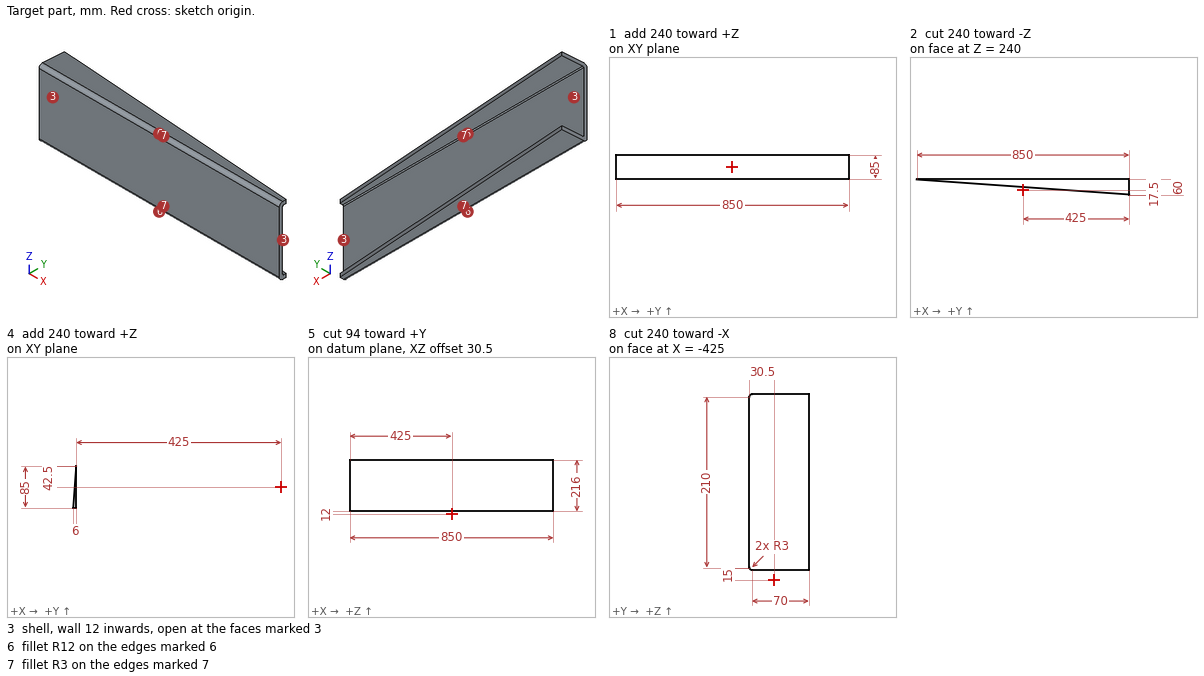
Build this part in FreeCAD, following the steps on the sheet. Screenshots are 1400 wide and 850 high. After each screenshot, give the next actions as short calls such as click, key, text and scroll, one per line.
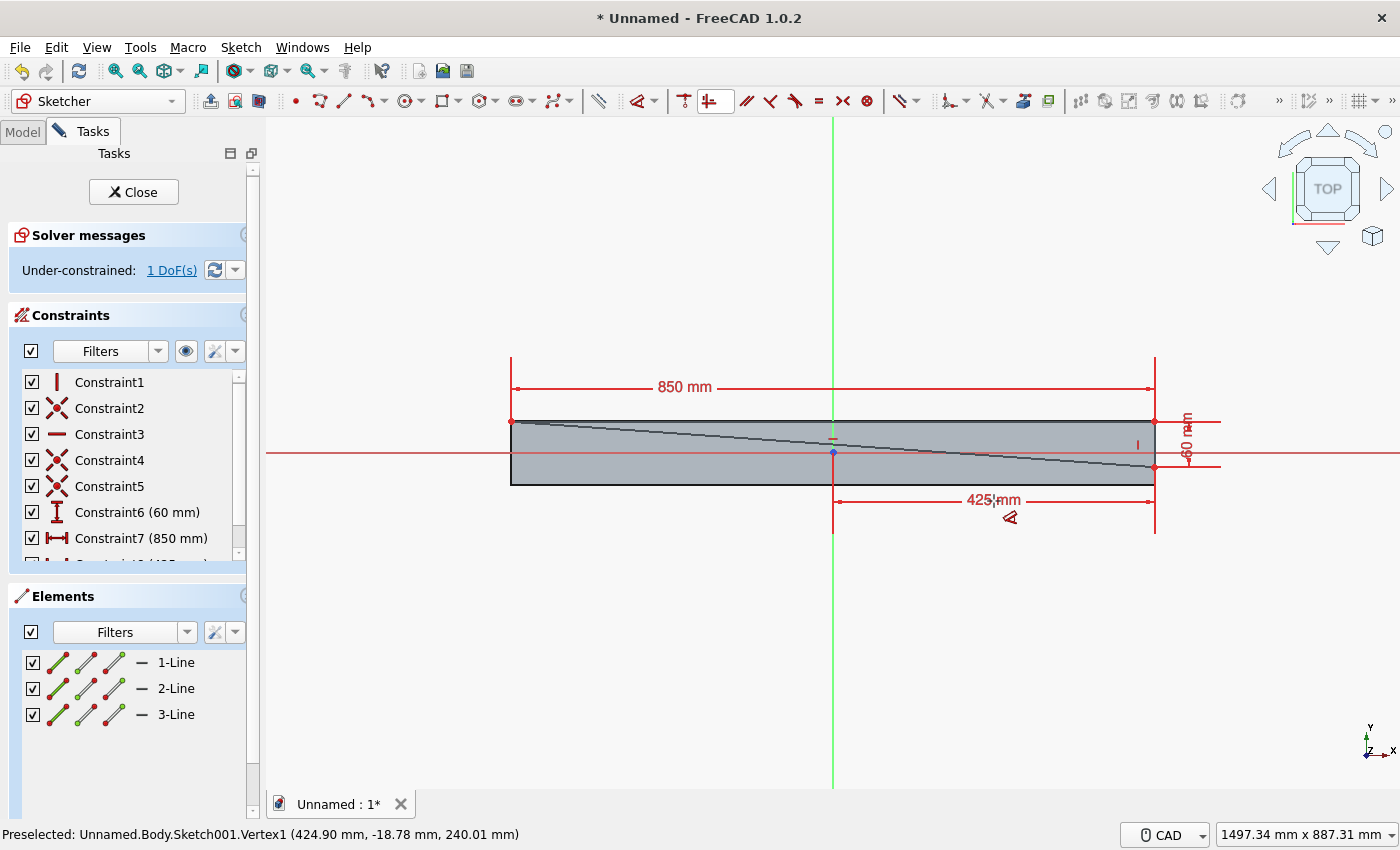
scroll(1155, 467, up, 6)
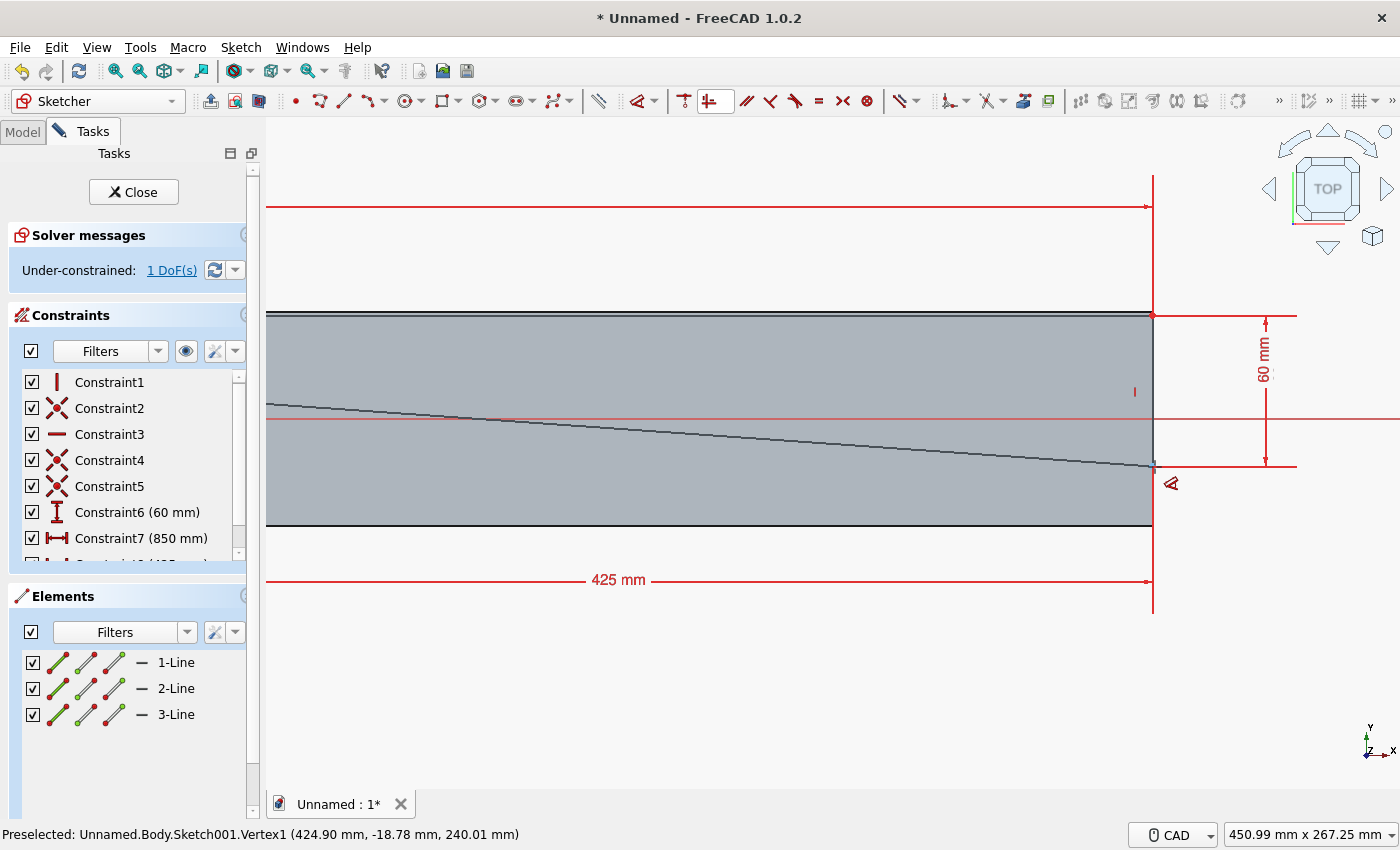
click(1153, 467)
click(1187, 443)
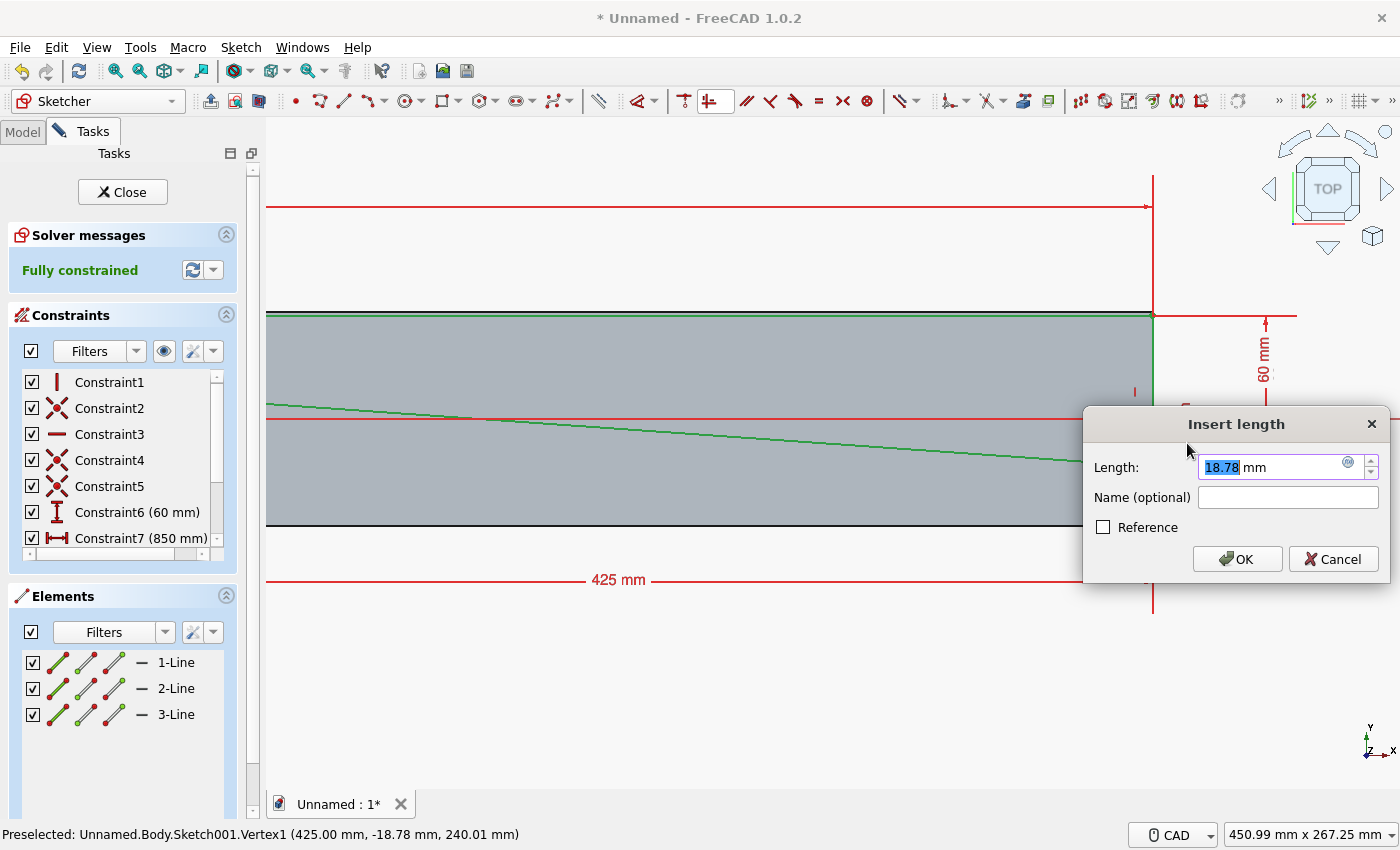
text(17.5)
key(Return)
key(Escape)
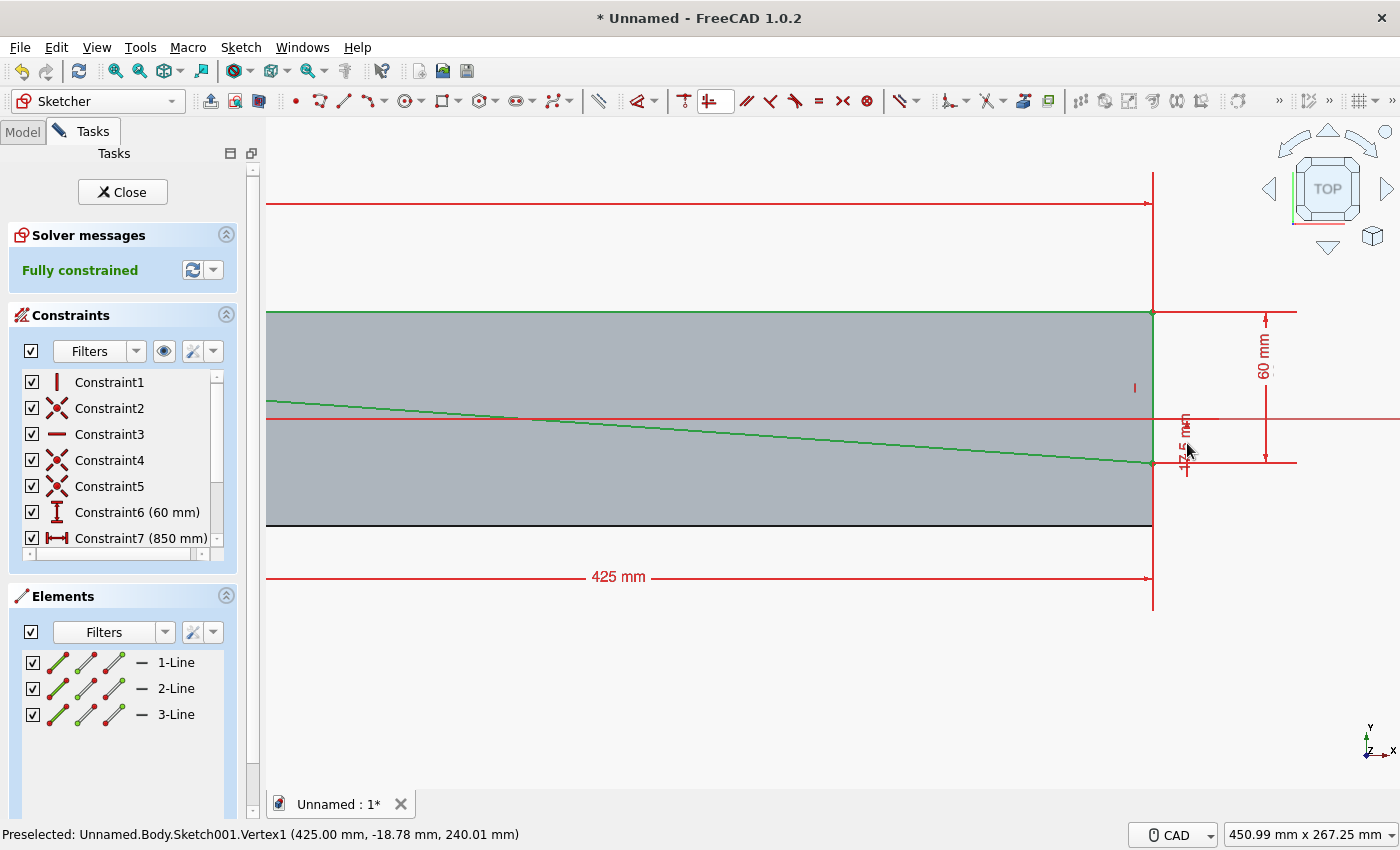
click(123, 192)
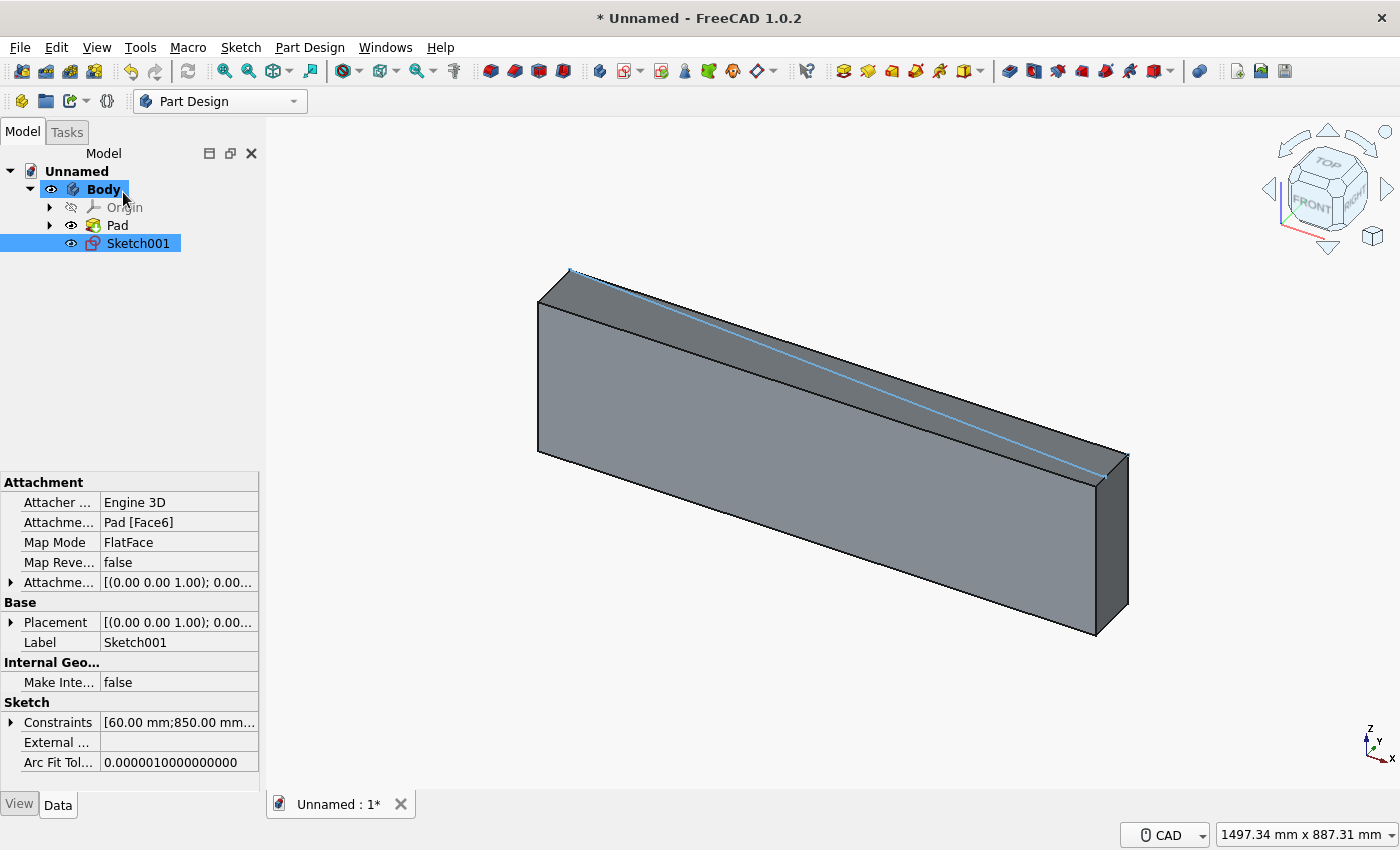
click(1010, 72)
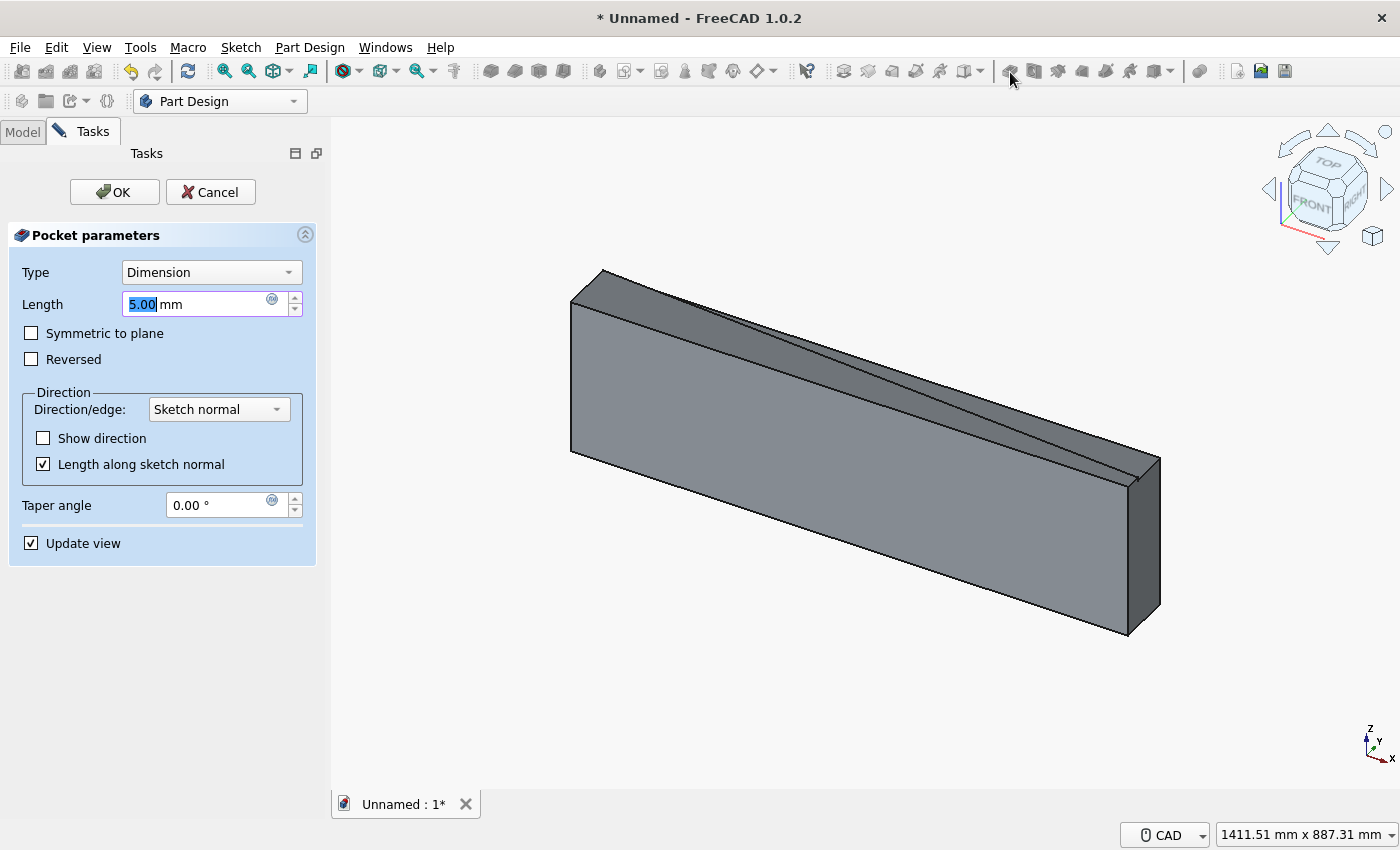
text(240)
key(Tab)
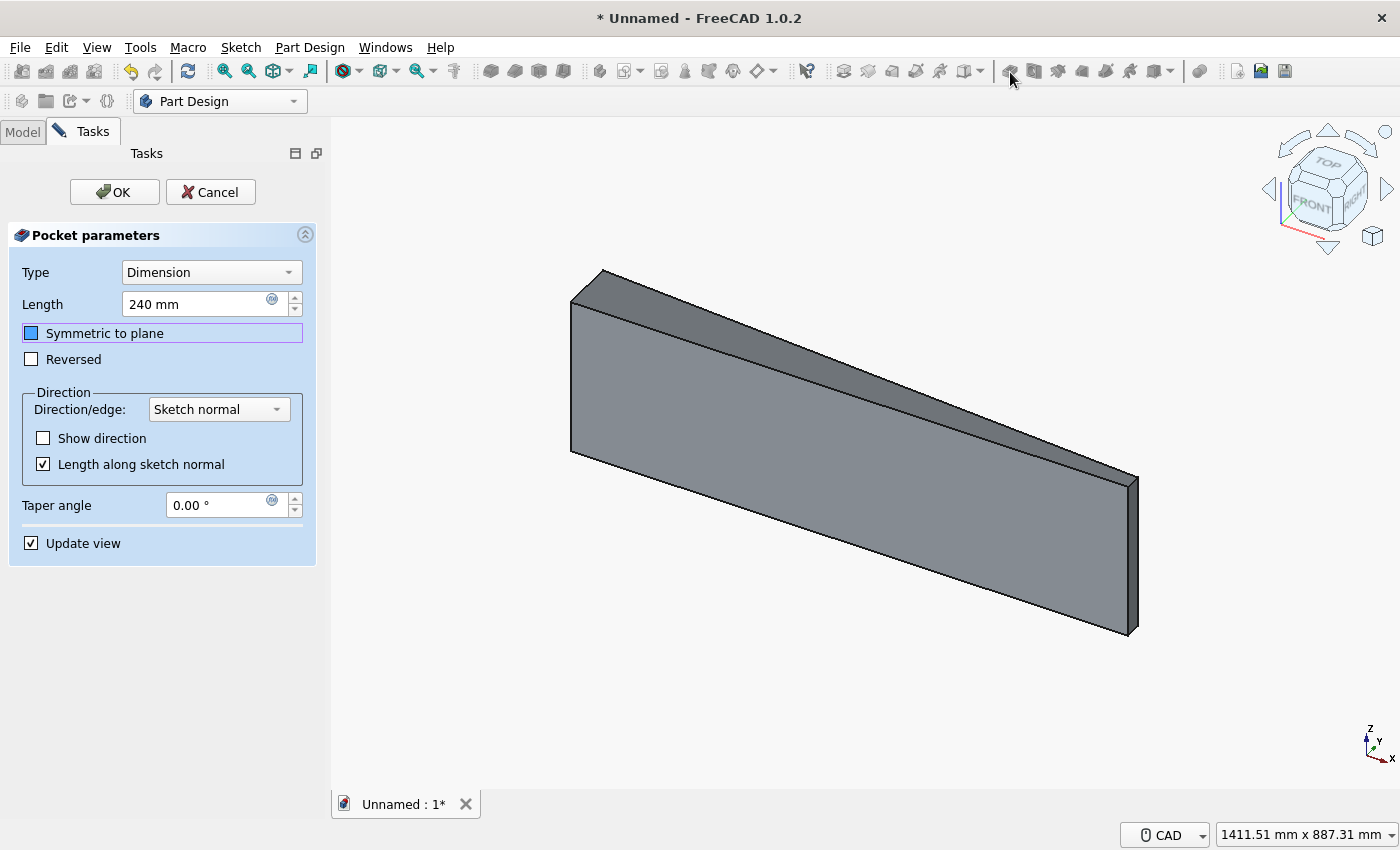
click(115, 192)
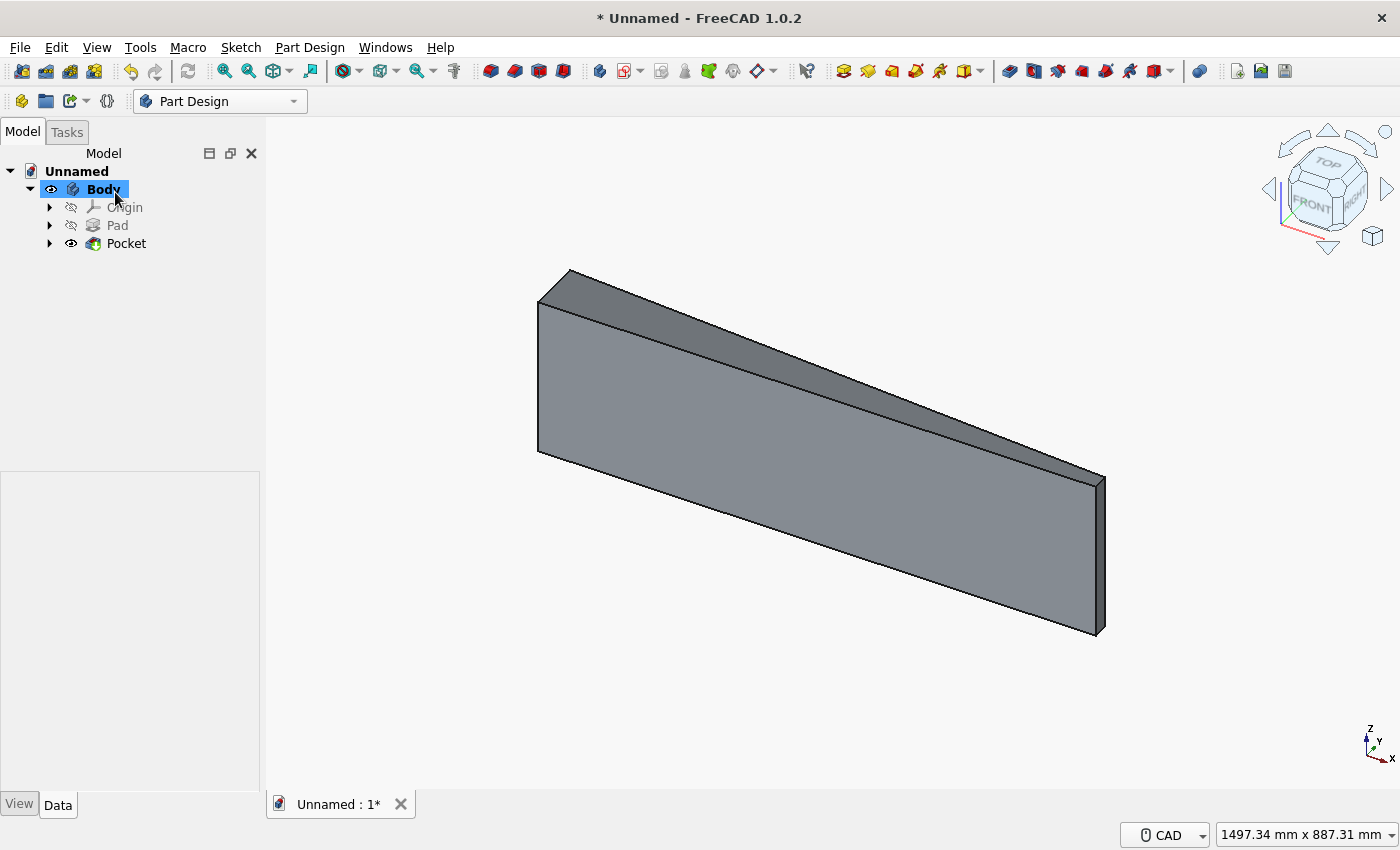
key(0)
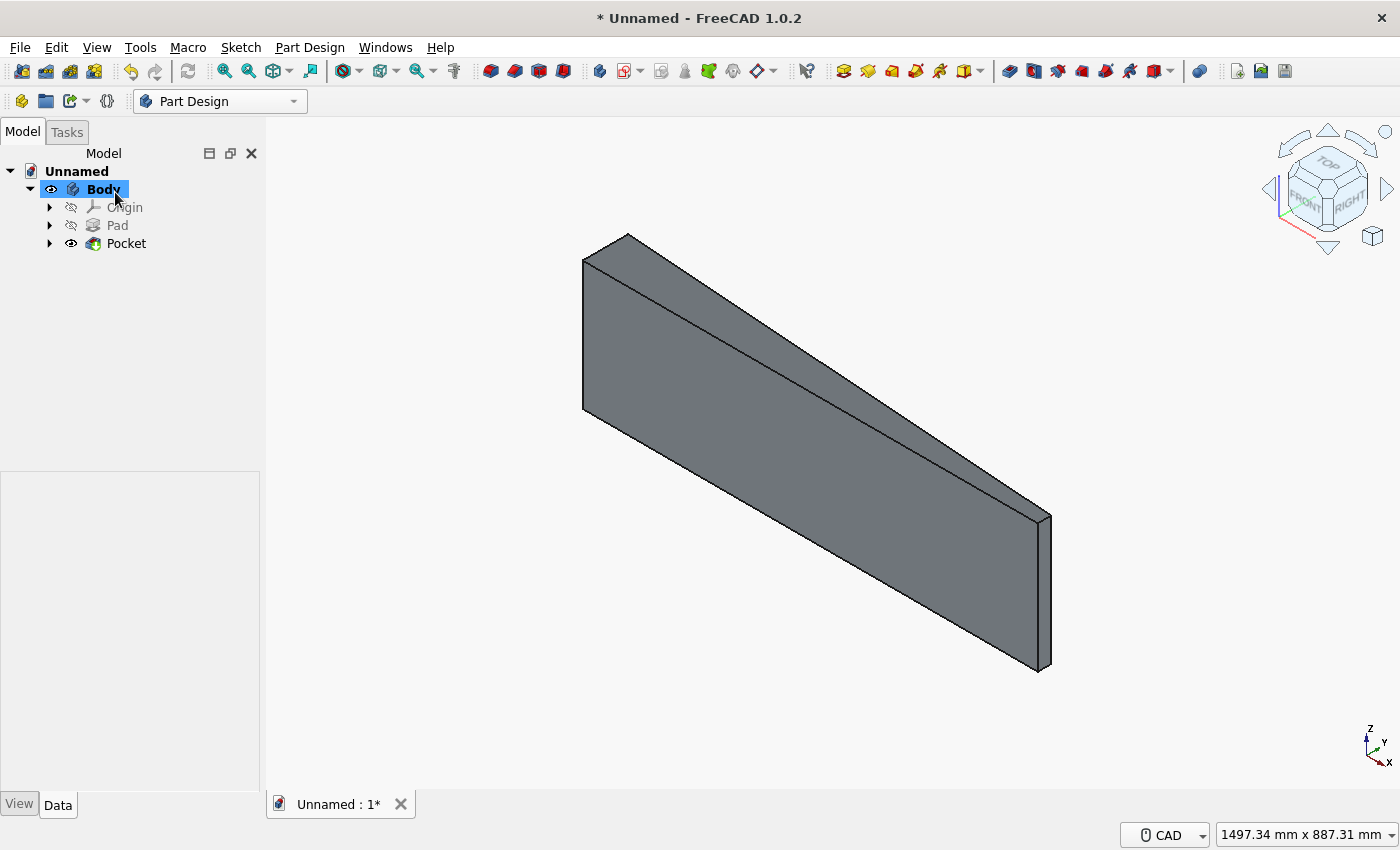
key(2)